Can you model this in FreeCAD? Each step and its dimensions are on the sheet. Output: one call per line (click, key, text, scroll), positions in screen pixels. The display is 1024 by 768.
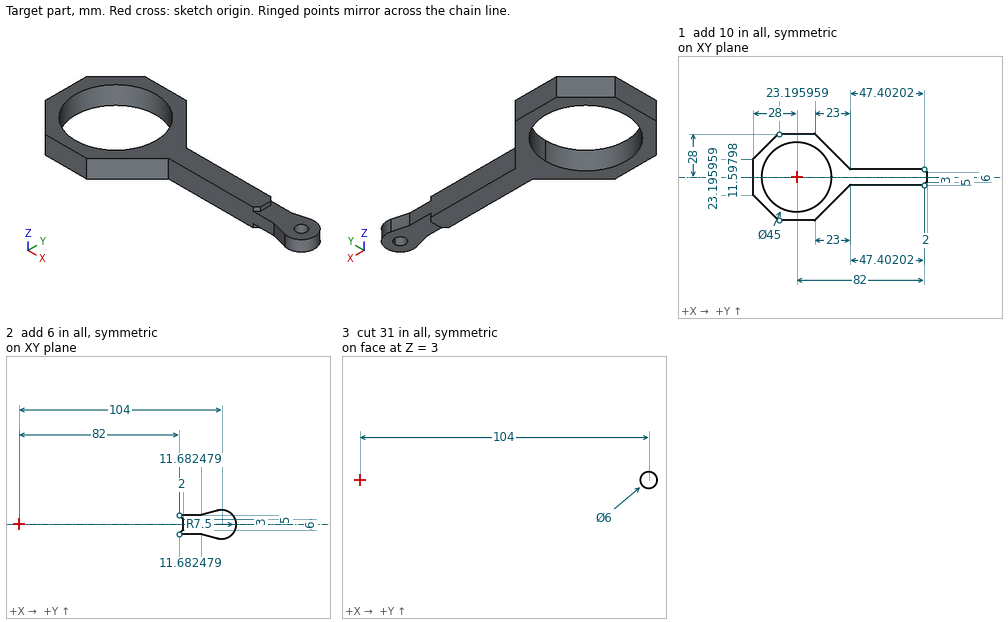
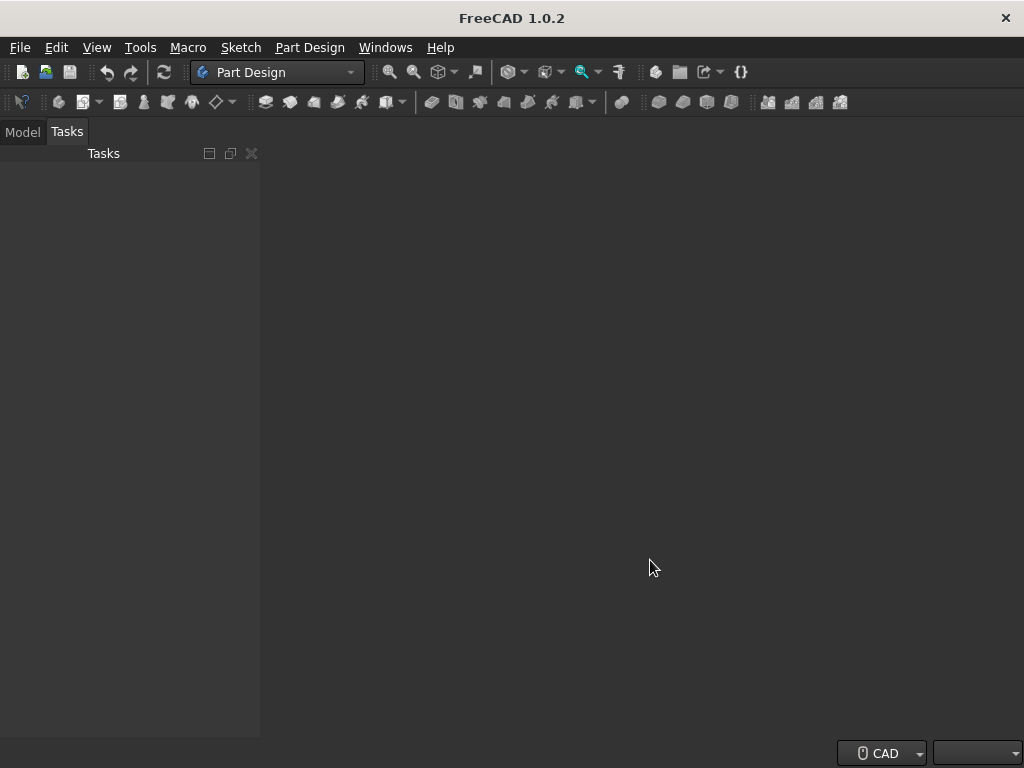
click(22, 72)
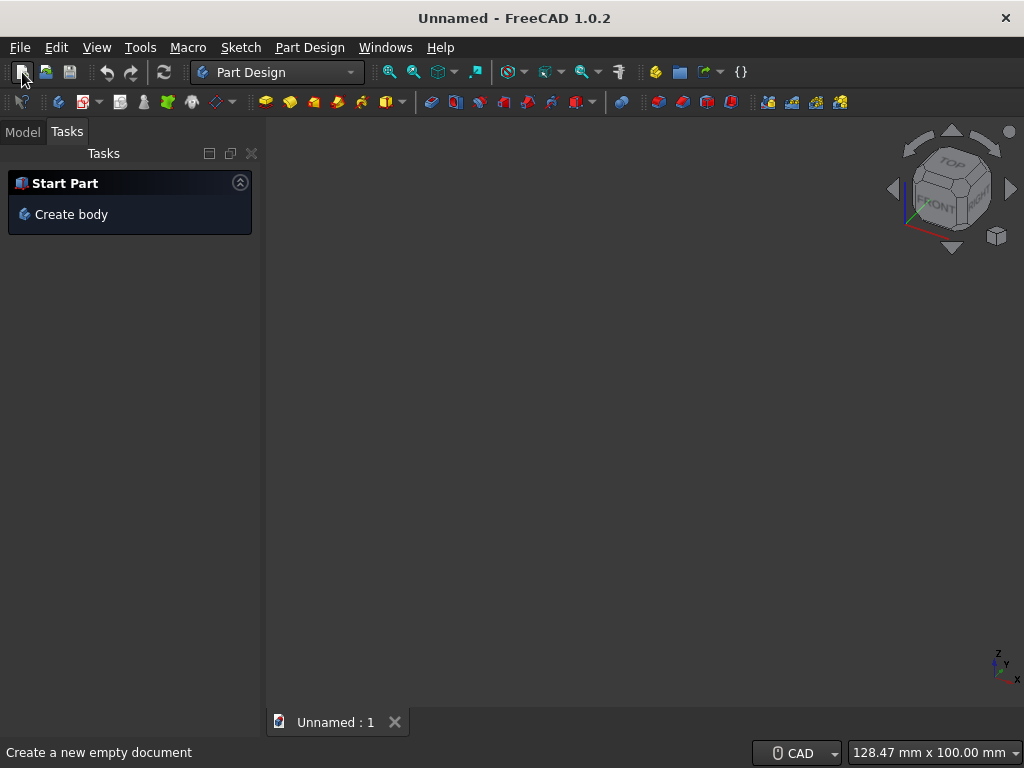
click(84, 102)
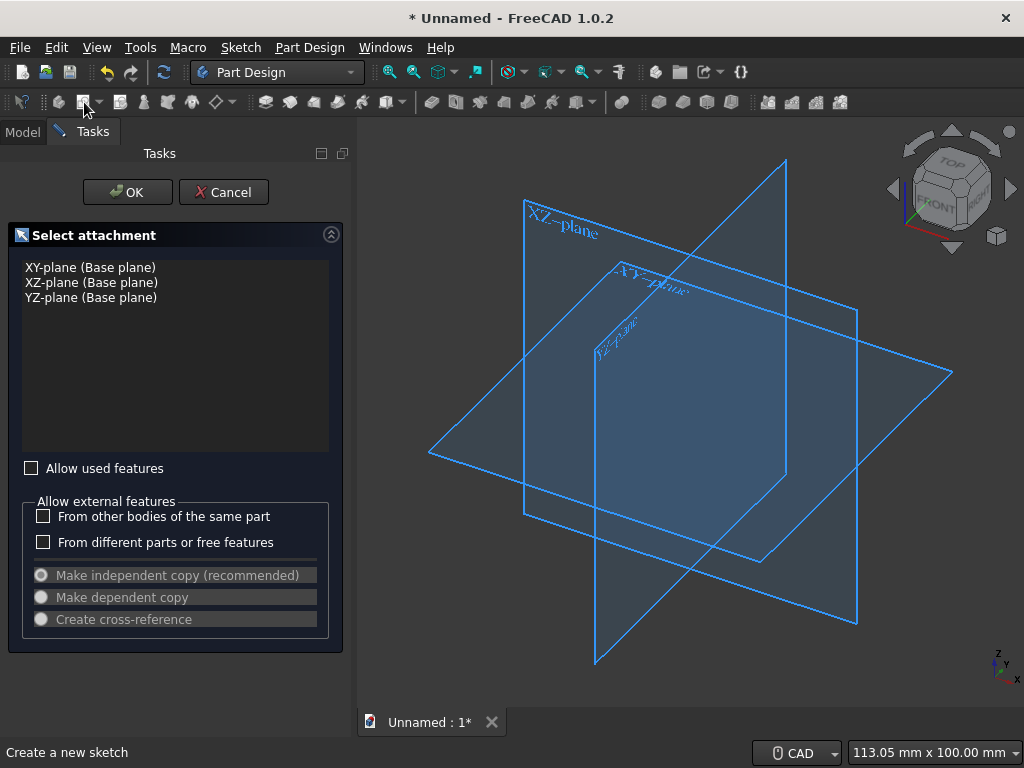
click(82, 268)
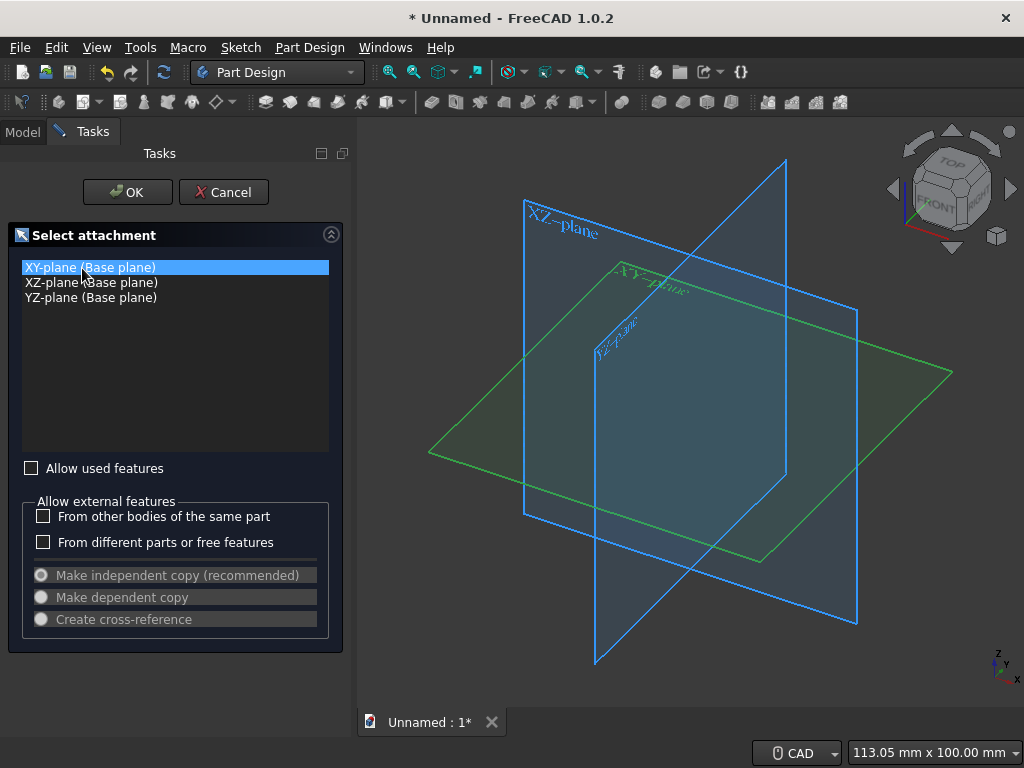
click(128, 192)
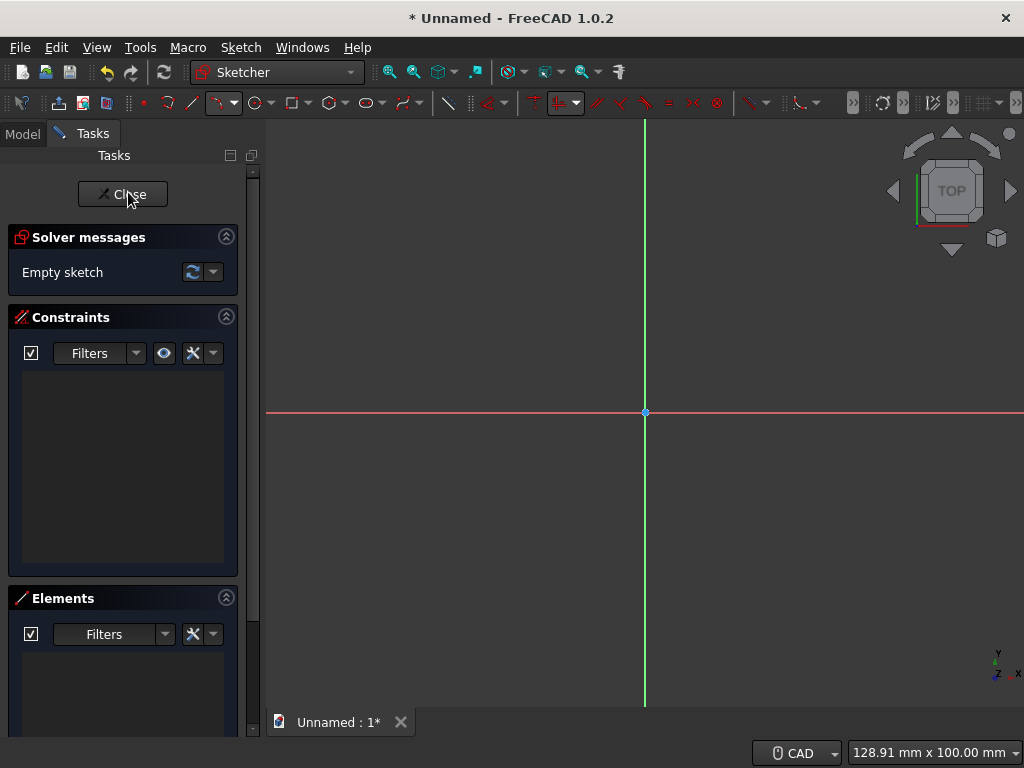
scroll(294, 413, down, 3)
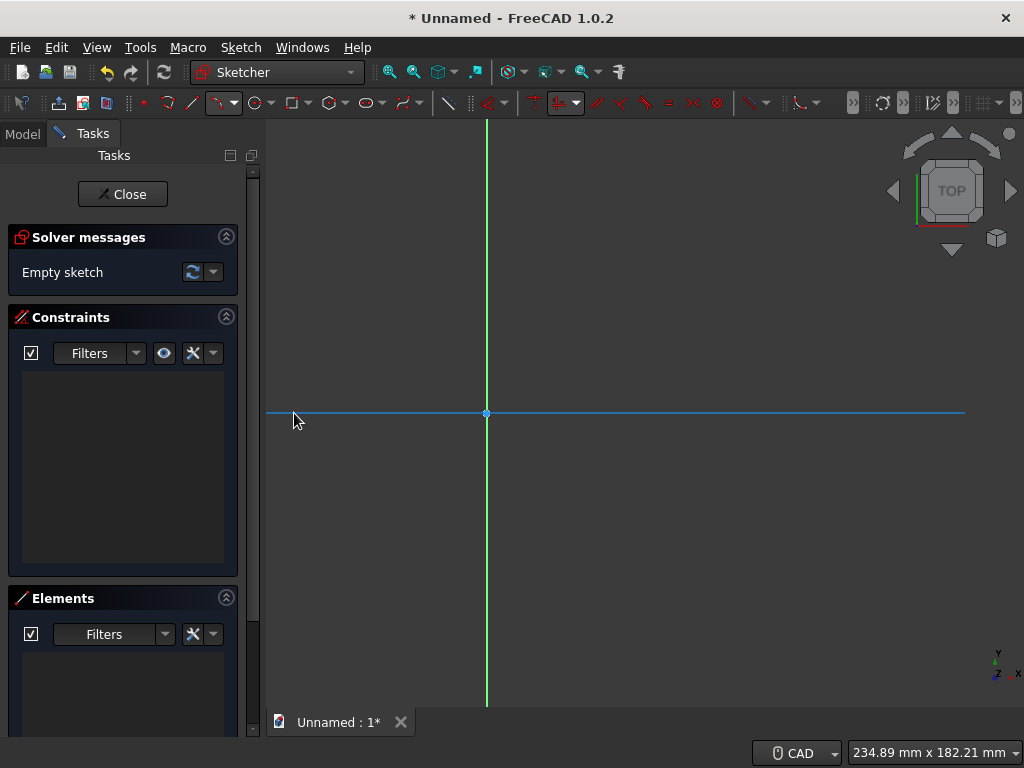
click(168, 104)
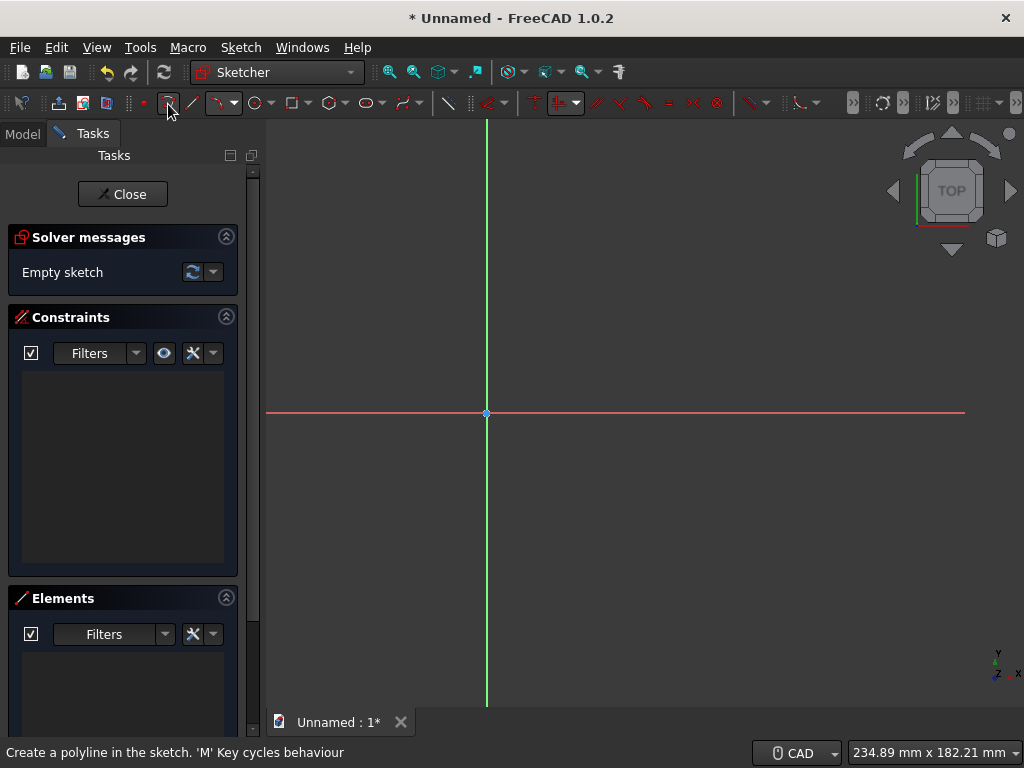
click(524, 323)
click(449, 323)
click(396, 376)
click(396, 451)
click(449, 504)
click(524, 504)
click(598, 429)
click(751, 429)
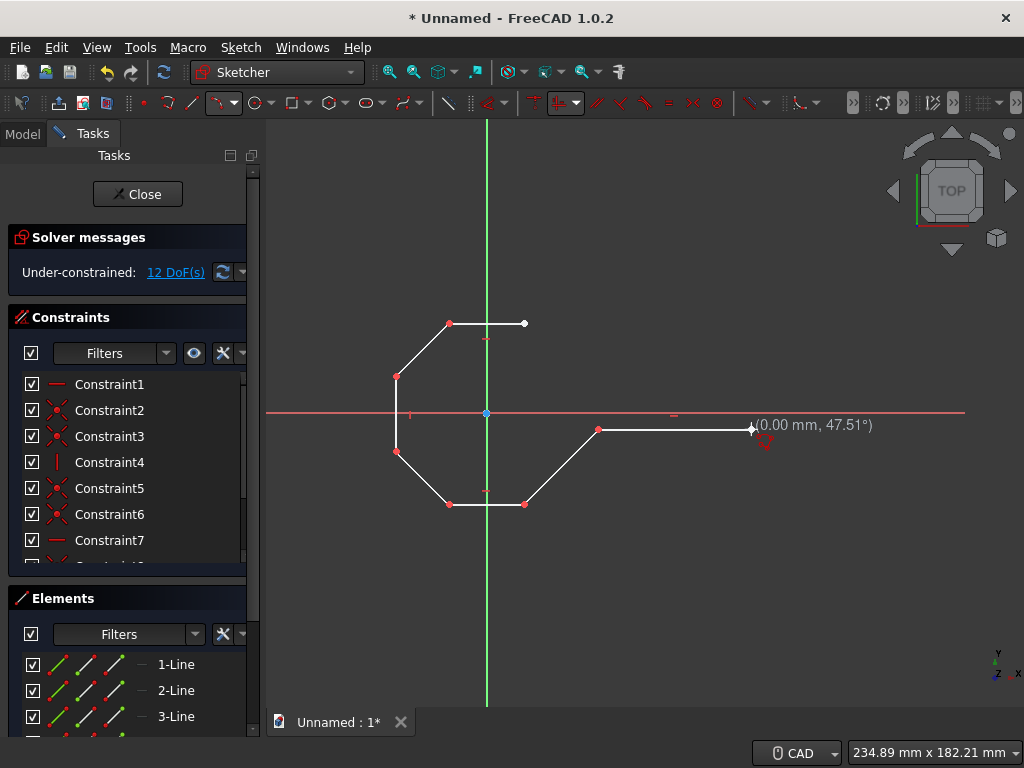
scroll(758, 423, up, 3)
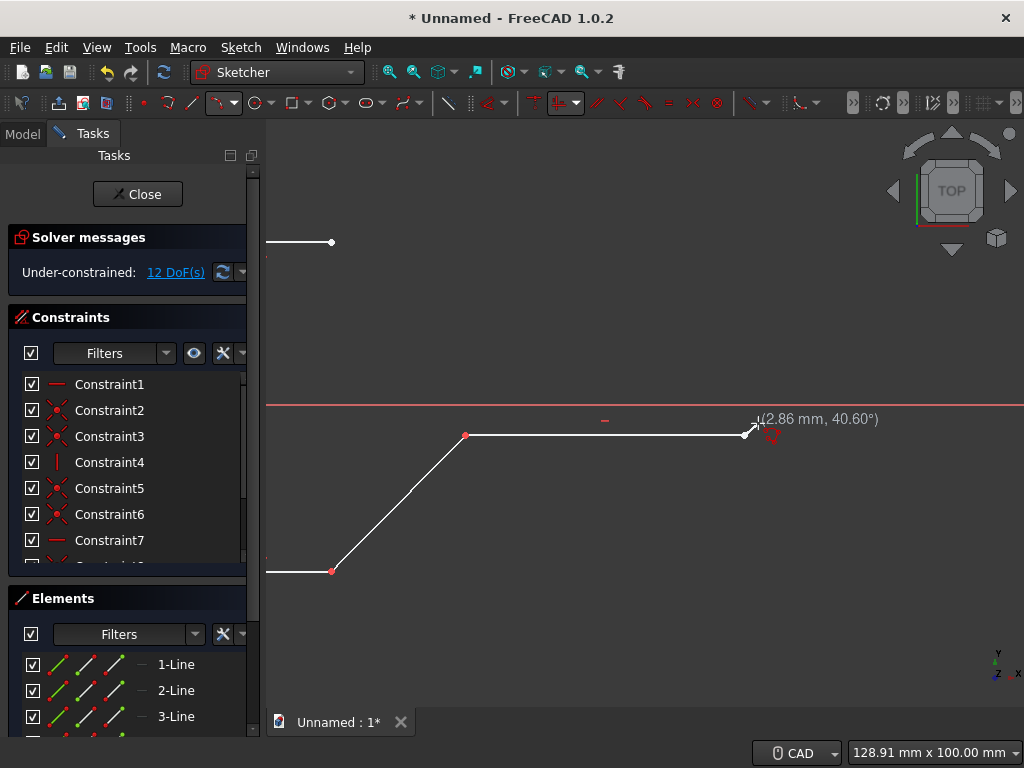
click(757, 422)
click(757, 387)
click(745, 375)
click(466, 375)
click(331, 242)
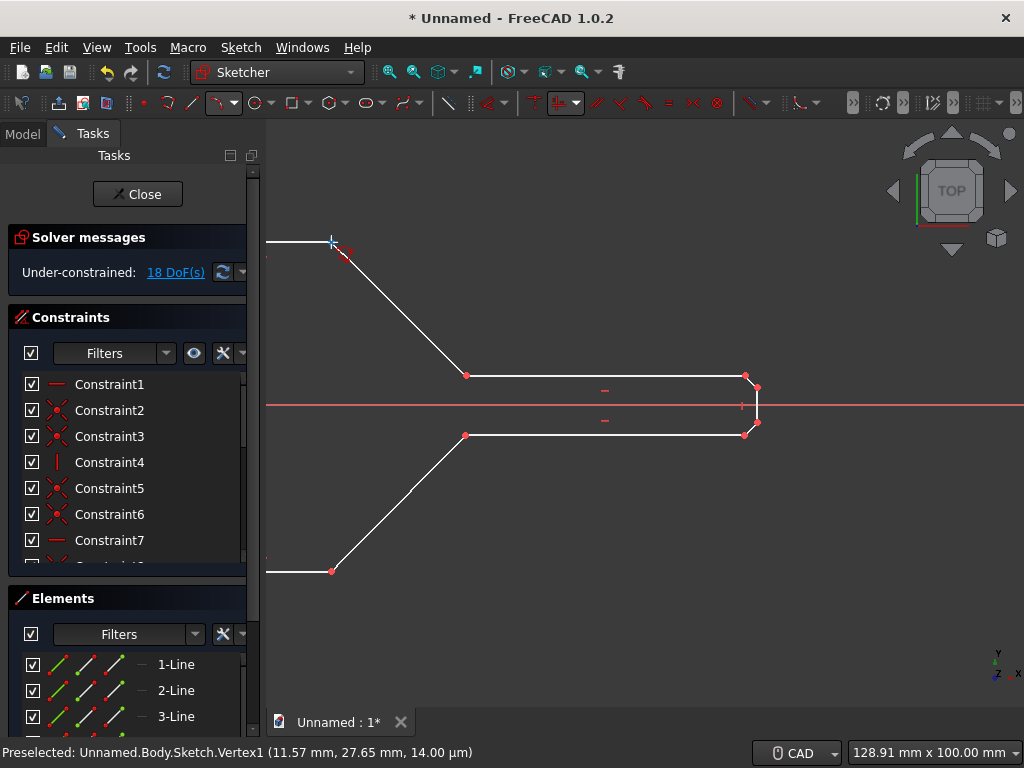
click(256, 104)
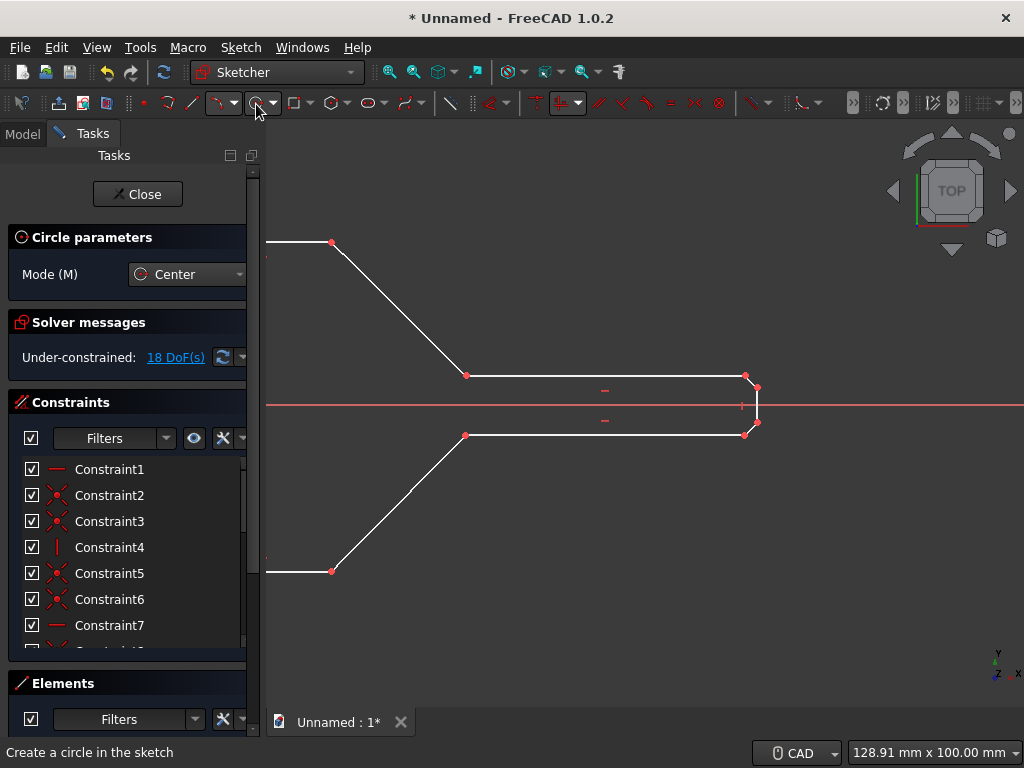
scroll(758, 423, down, 3)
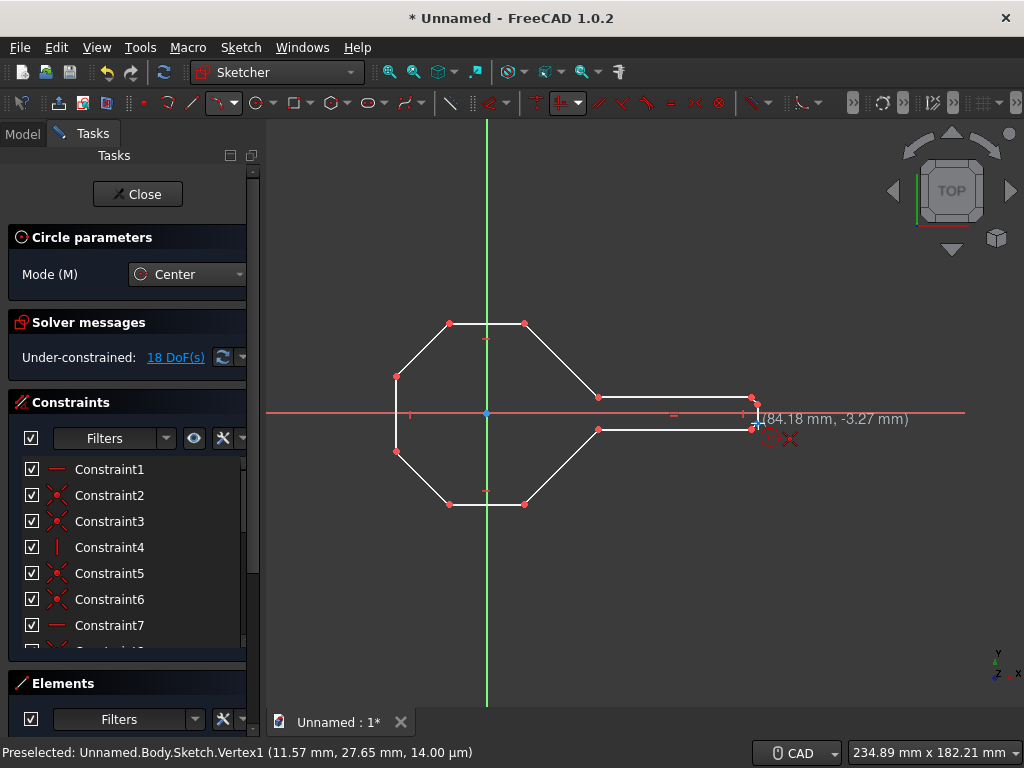
click(487, 413)
move(538, 362)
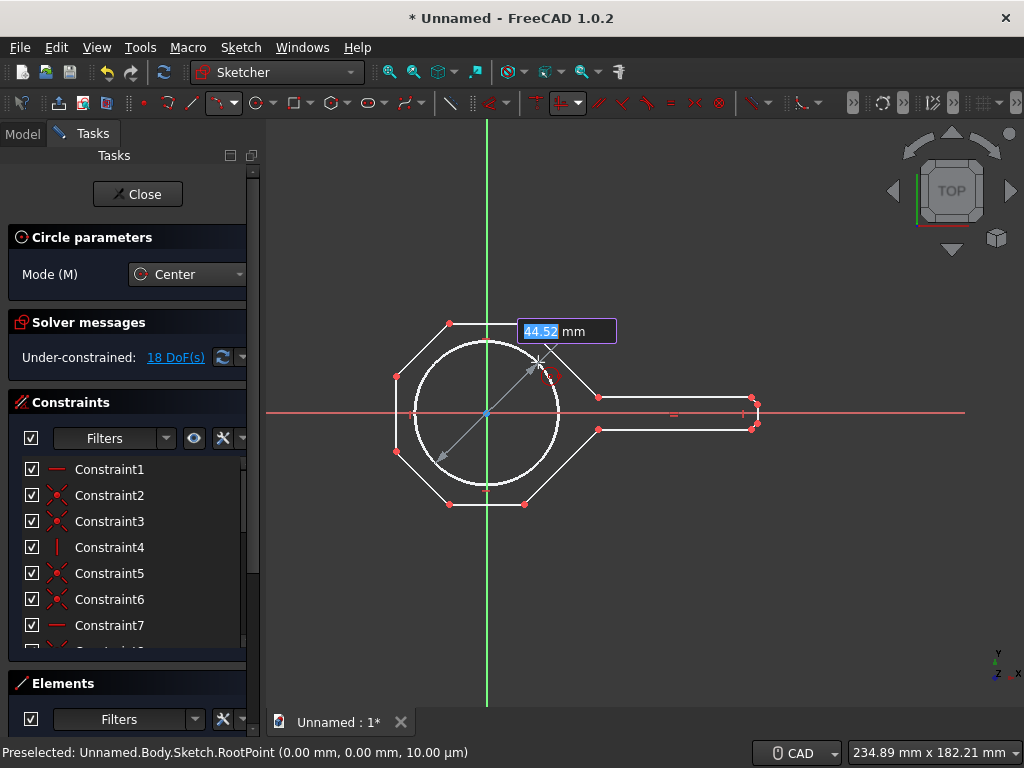
text(45)
key(Return)
key(Escape)